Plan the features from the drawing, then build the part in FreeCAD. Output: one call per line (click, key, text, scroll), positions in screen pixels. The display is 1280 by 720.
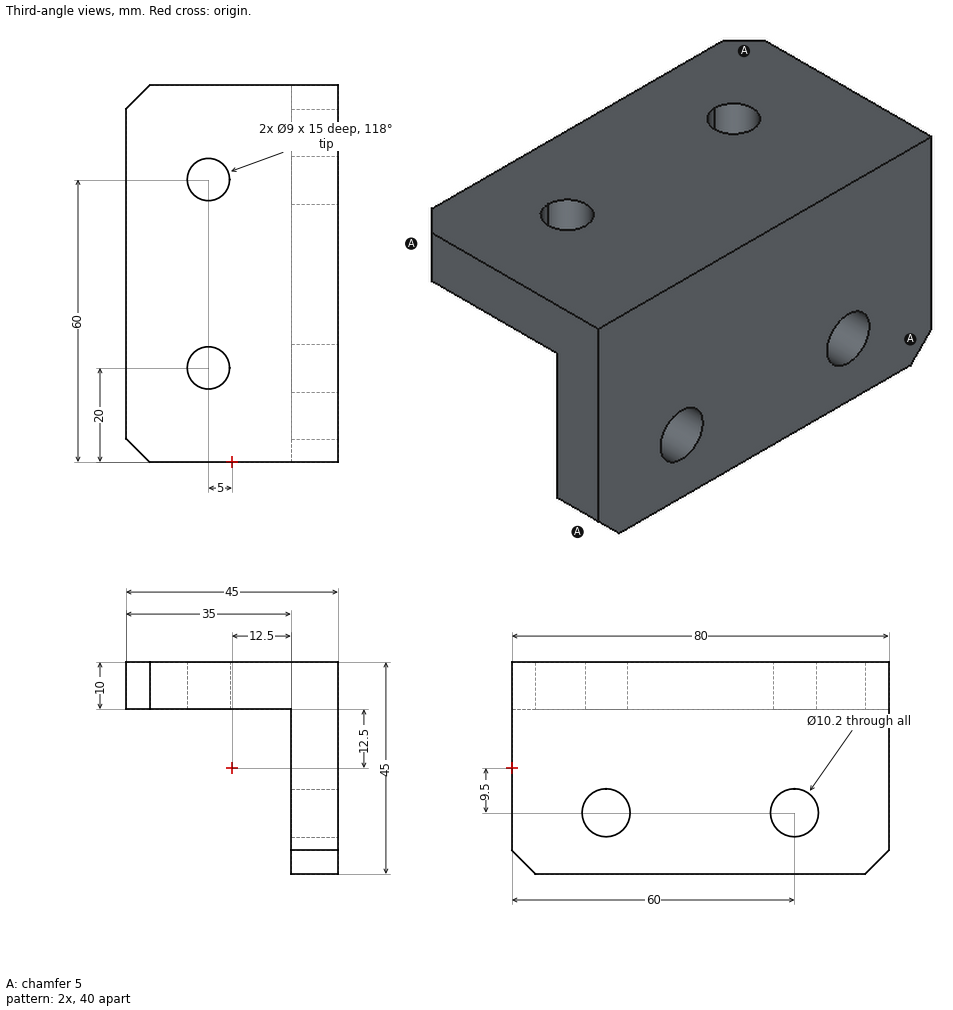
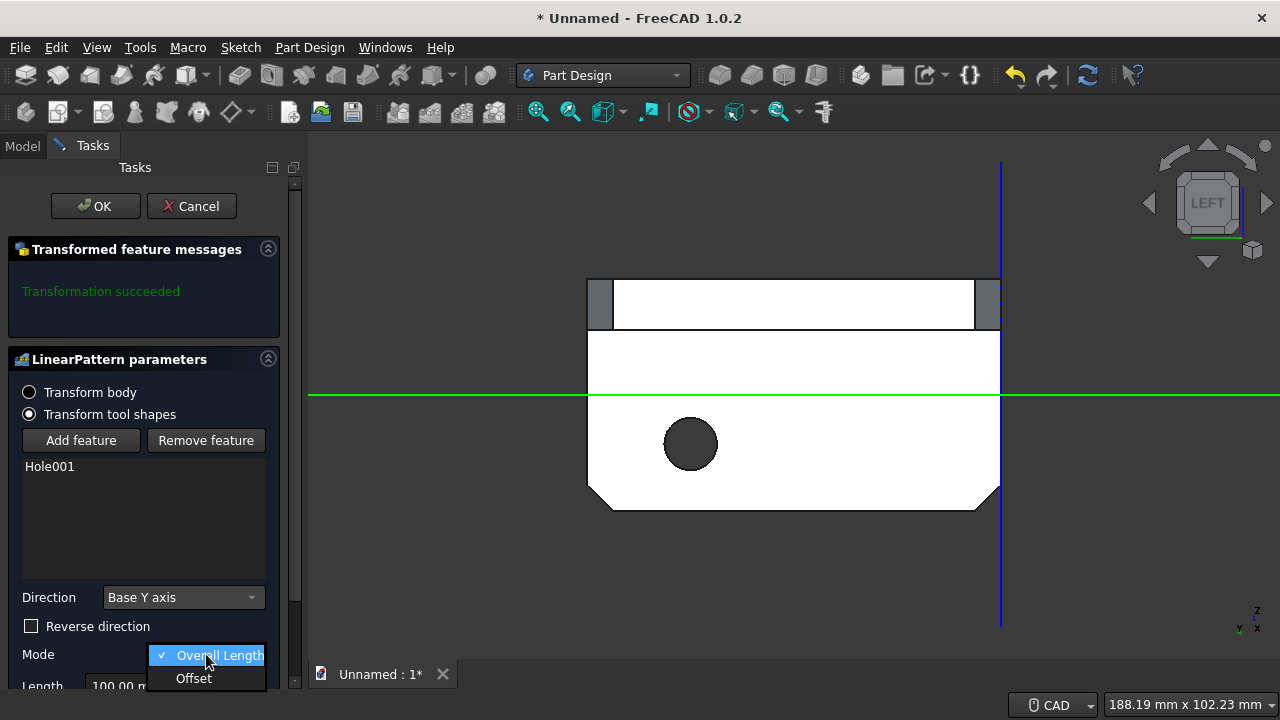
click(206, 678)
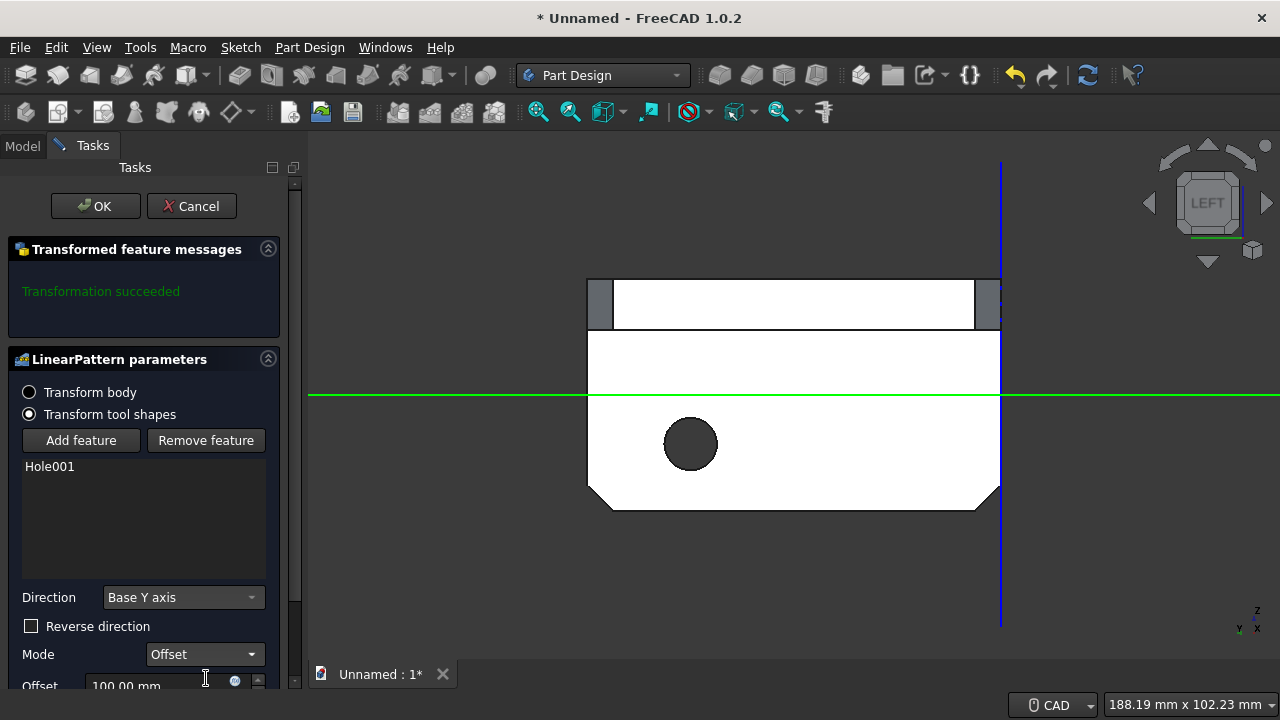
scroll(295, 432, down, 2)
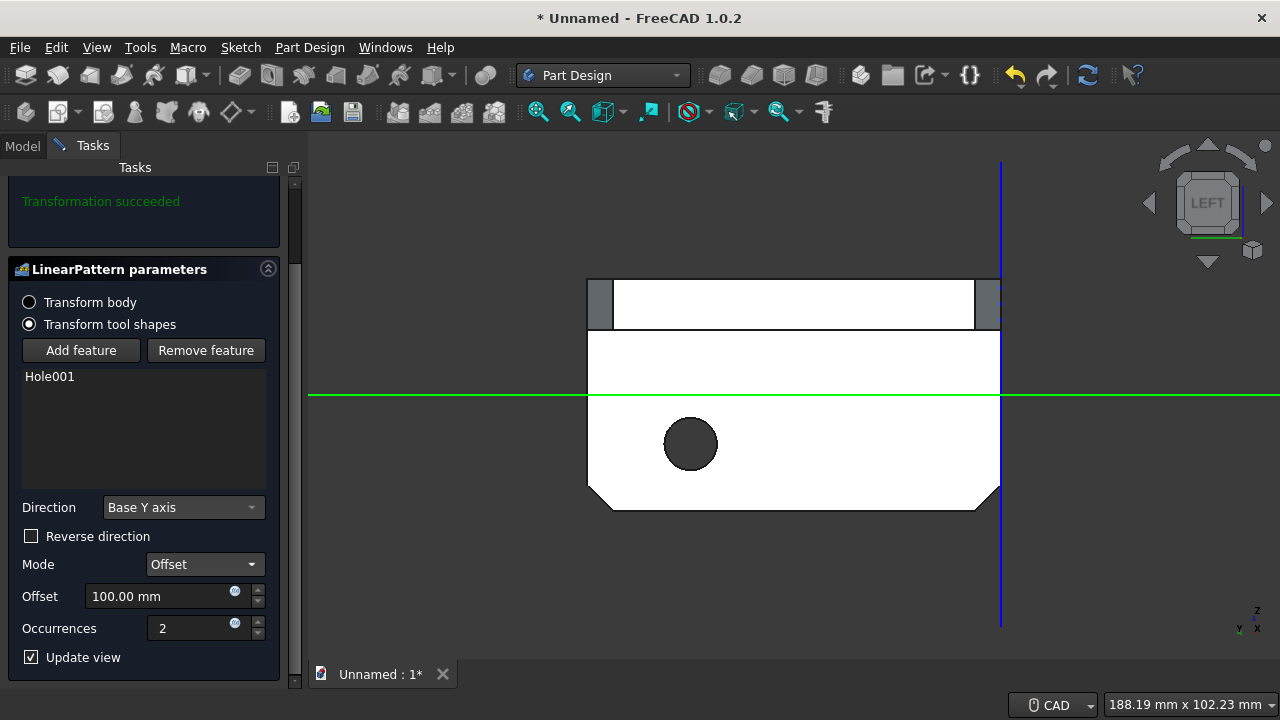
triple_click(168, 596)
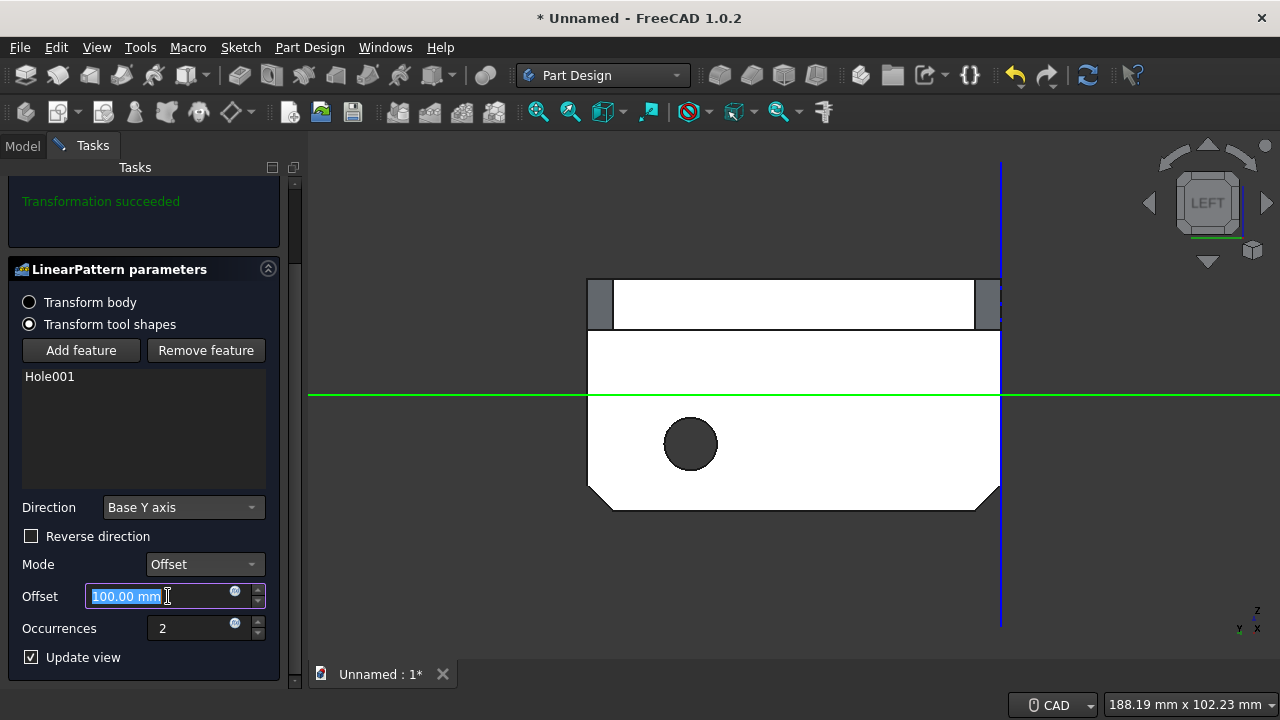
text(40)
key(Tab)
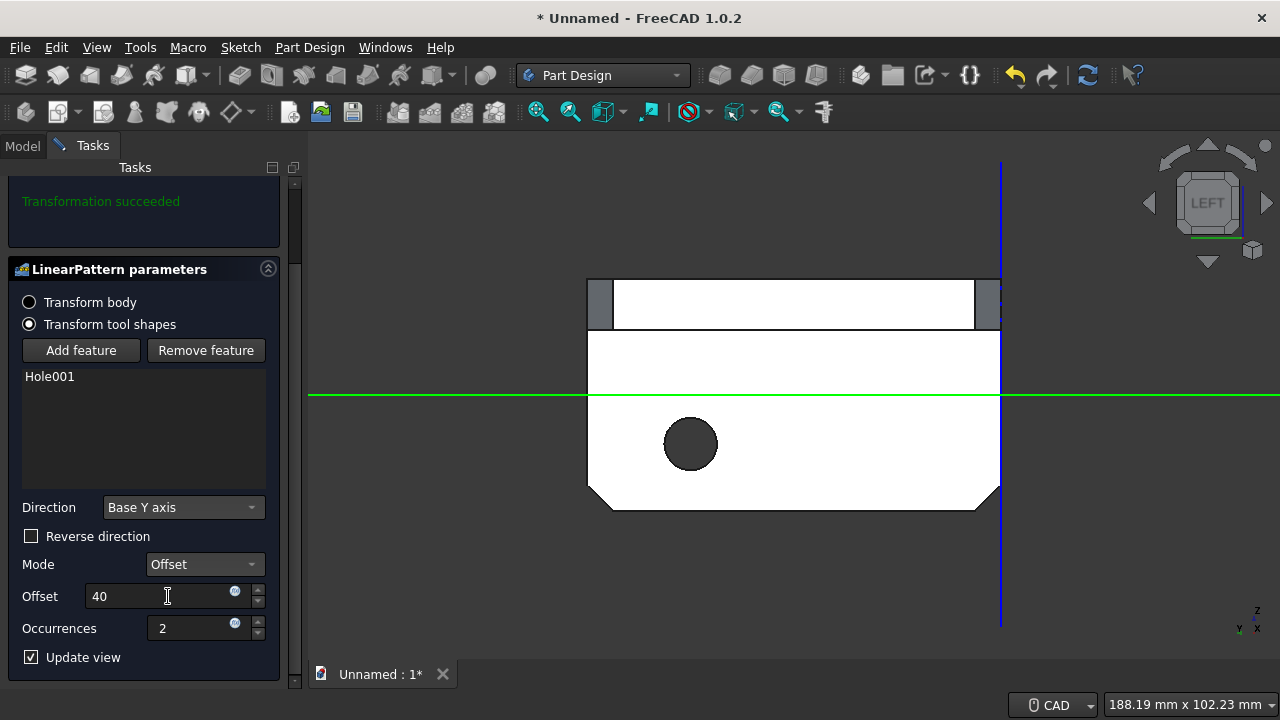
triple_click(198, 628)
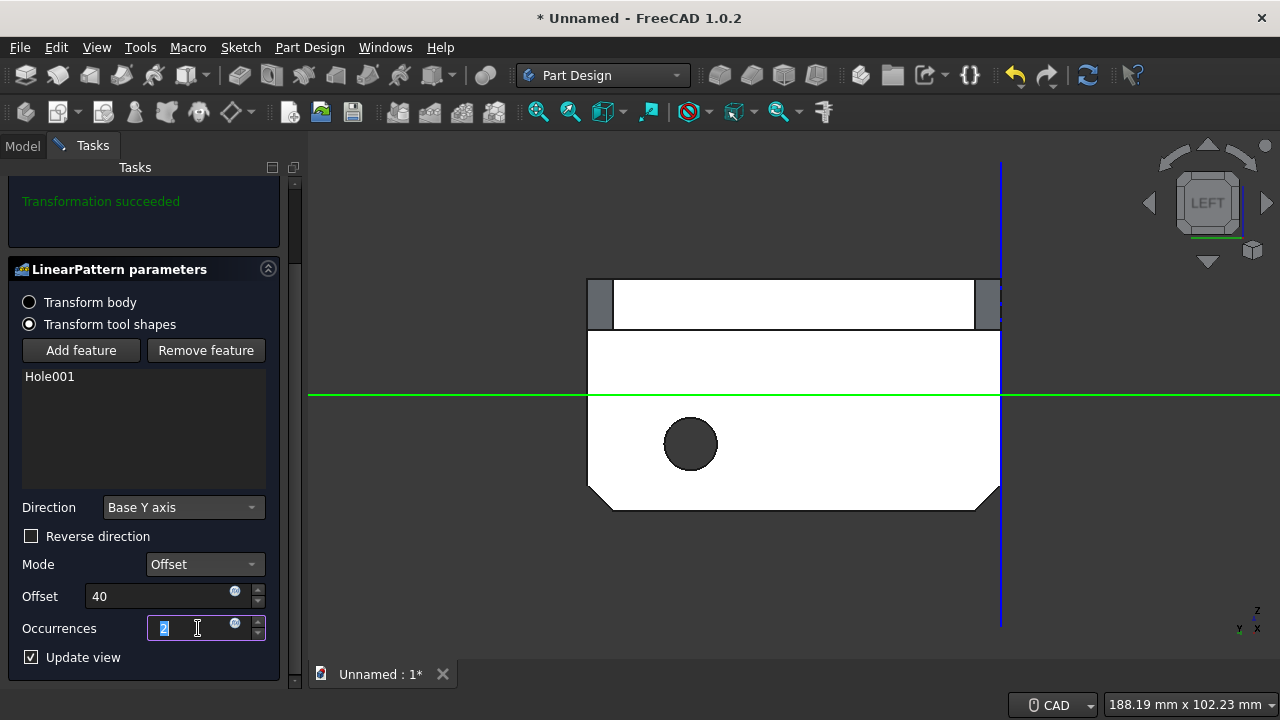
text(2)
key(Tab)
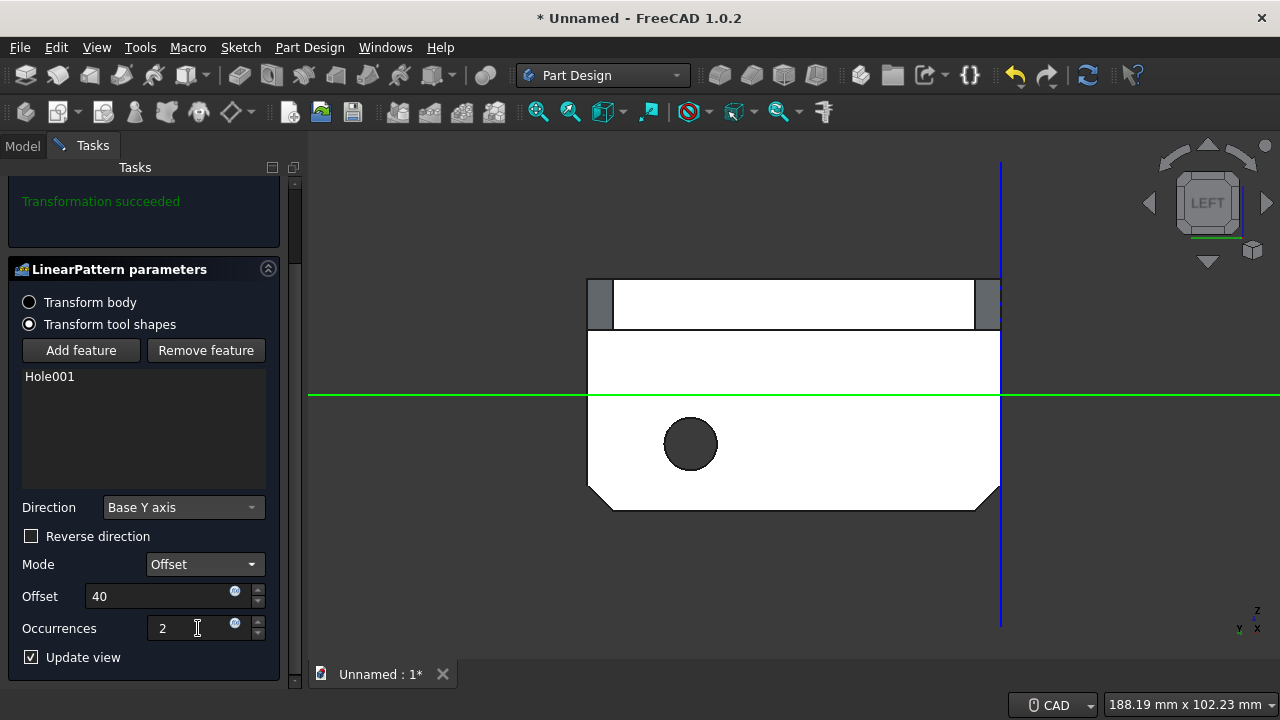
click(30, 536)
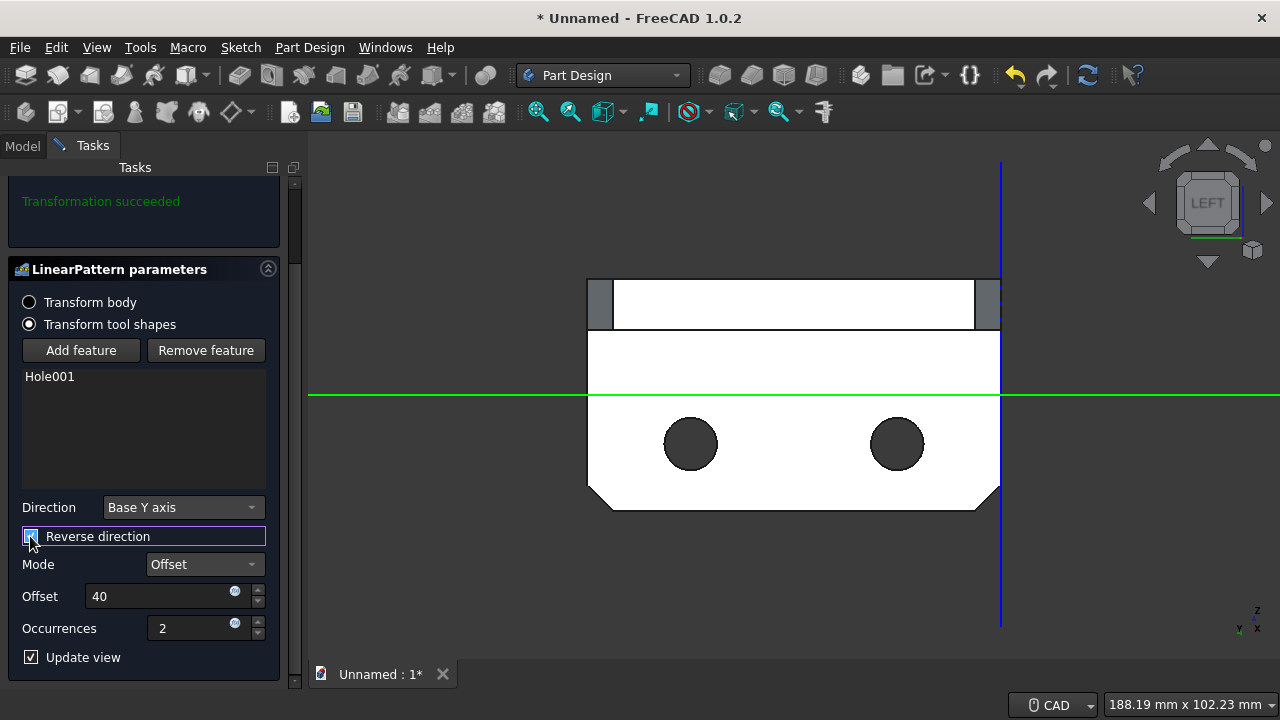
scroll(295, 432, up, 3)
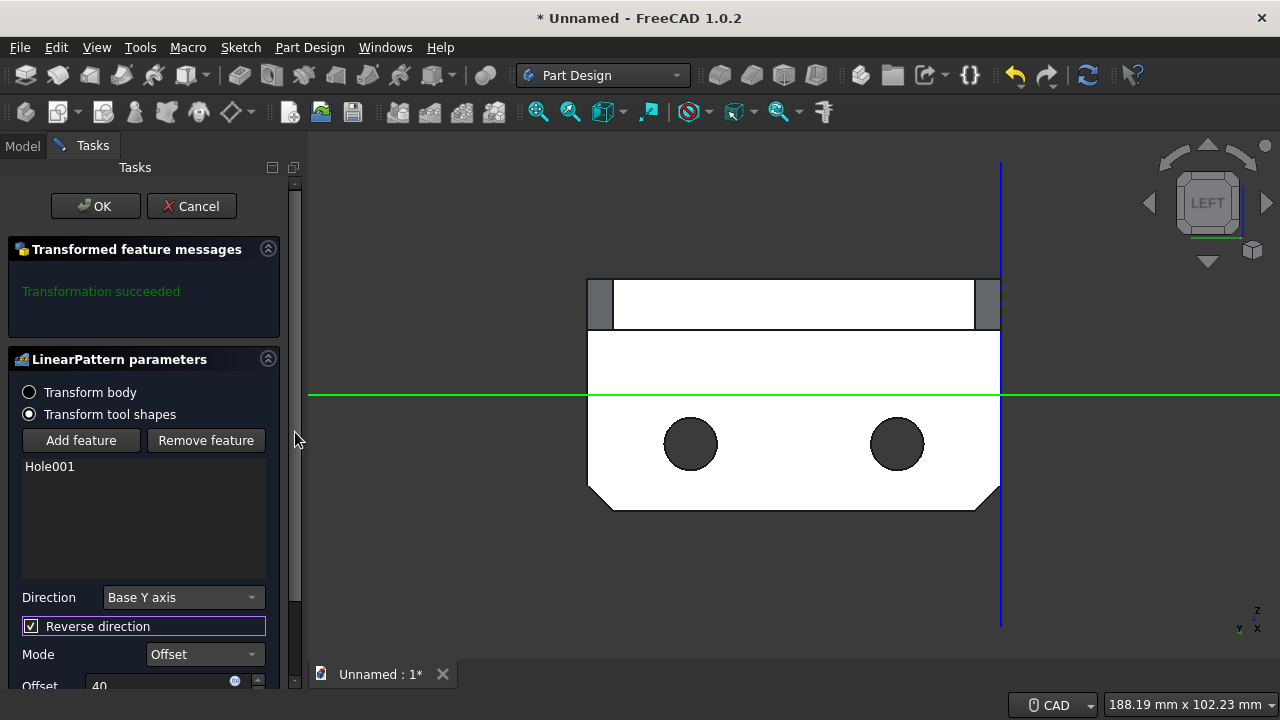
click(96, 206)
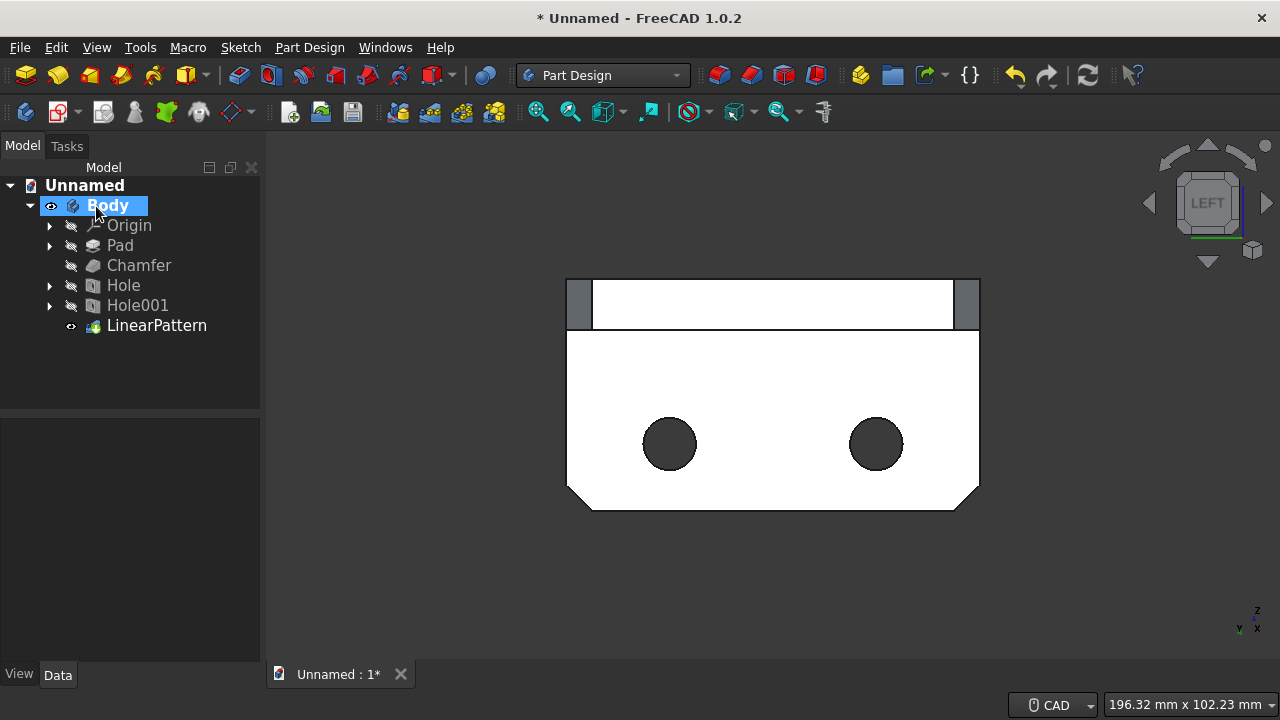
key(0)